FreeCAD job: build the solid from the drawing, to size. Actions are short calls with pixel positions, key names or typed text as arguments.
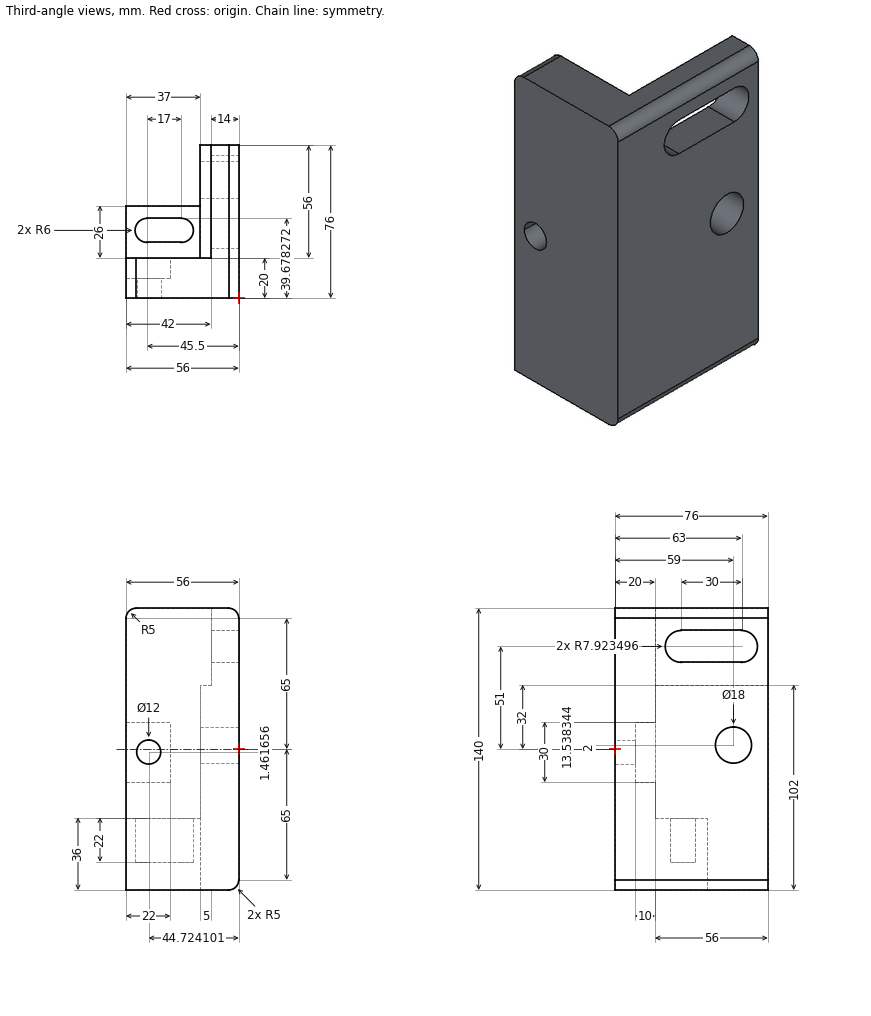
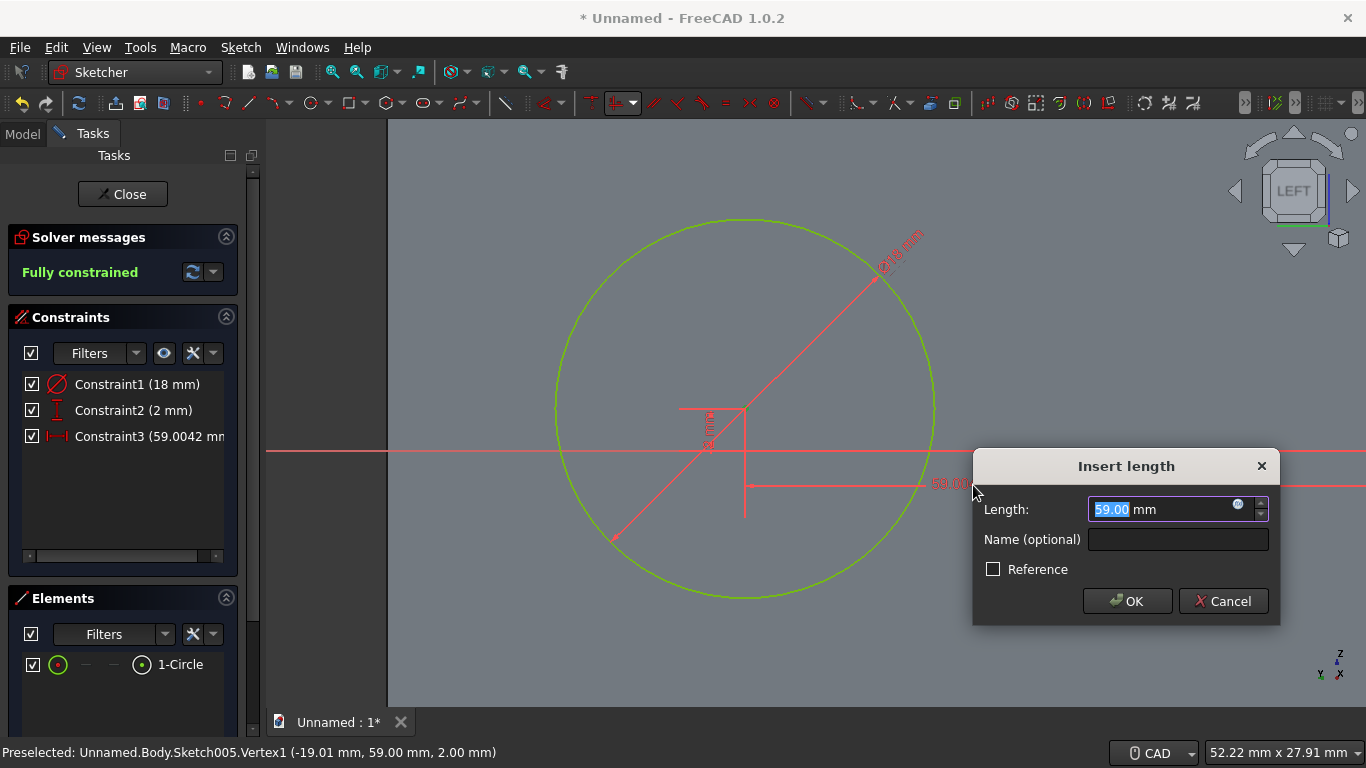
text(59)
key(Return)
key(Escape)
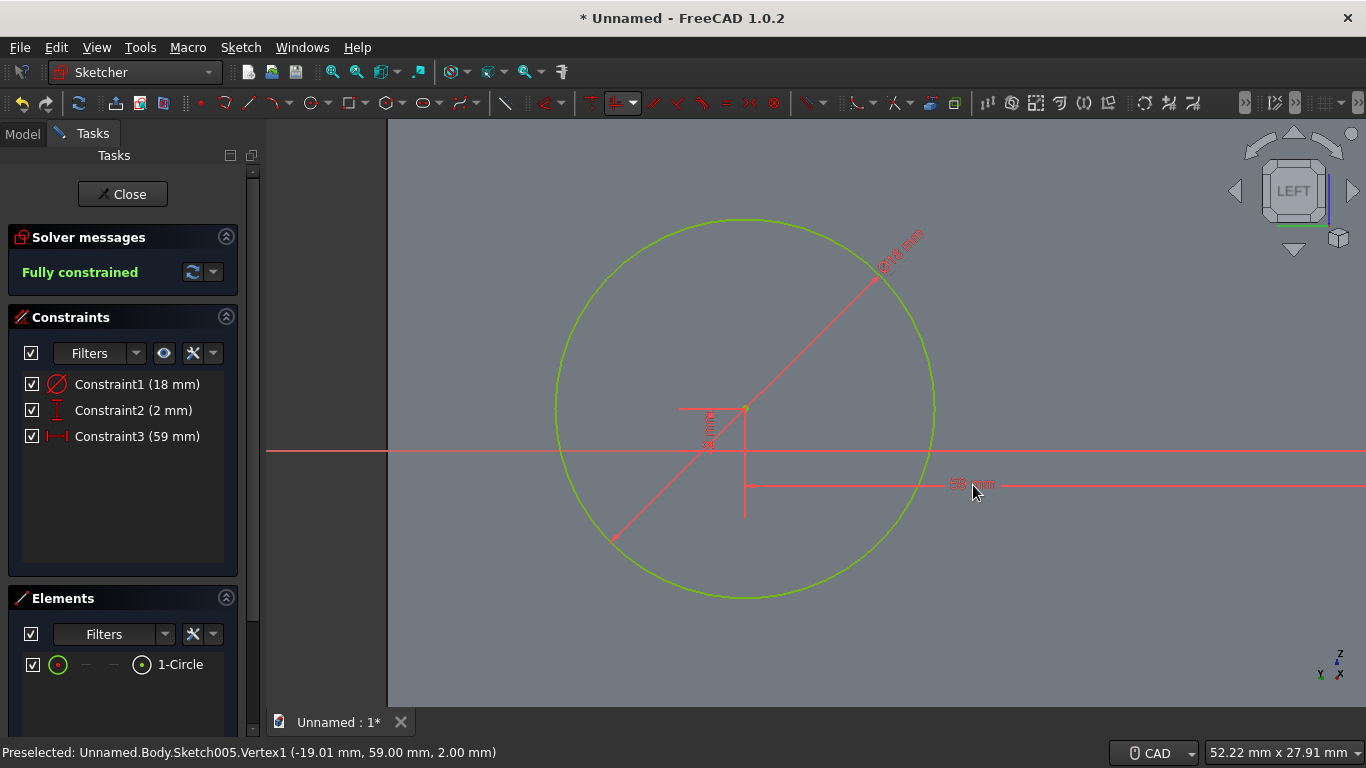
click(123, 194)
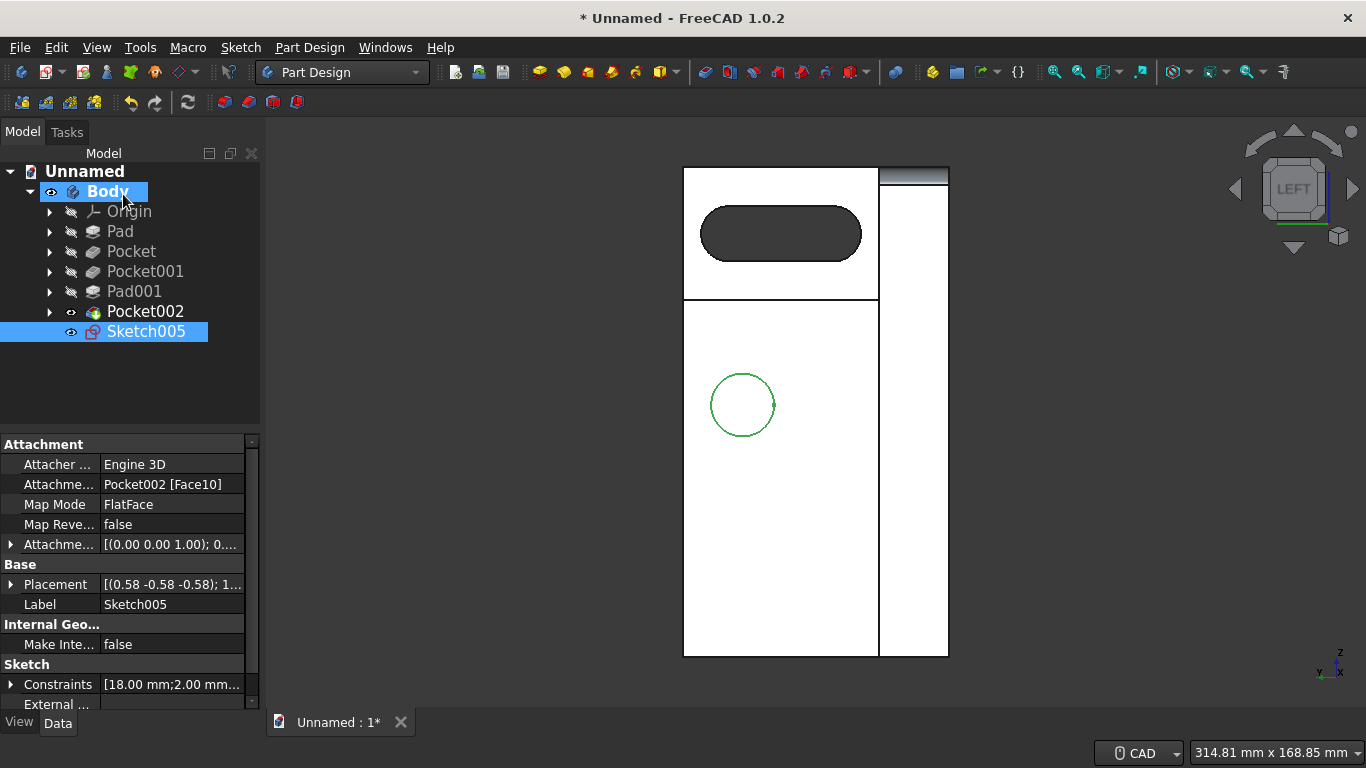
click(706, 72)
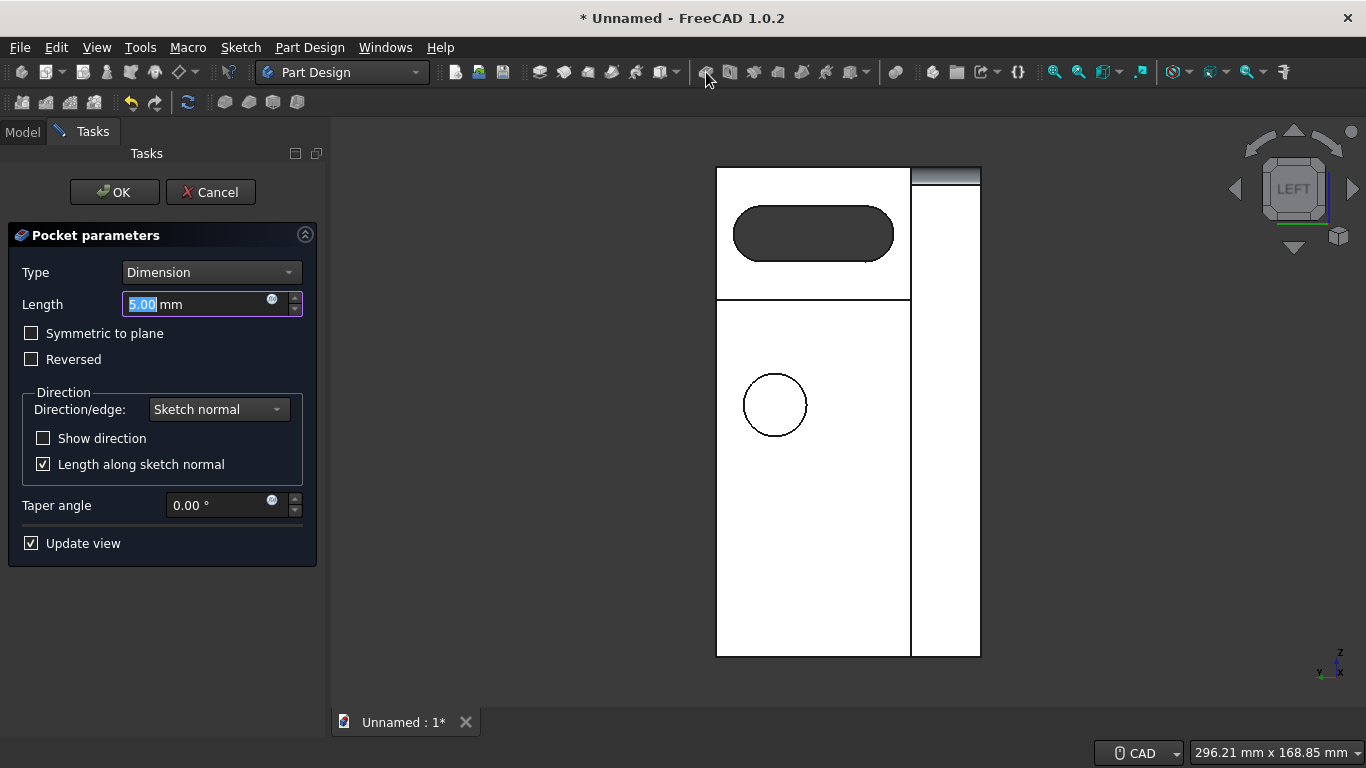
click(212, 272)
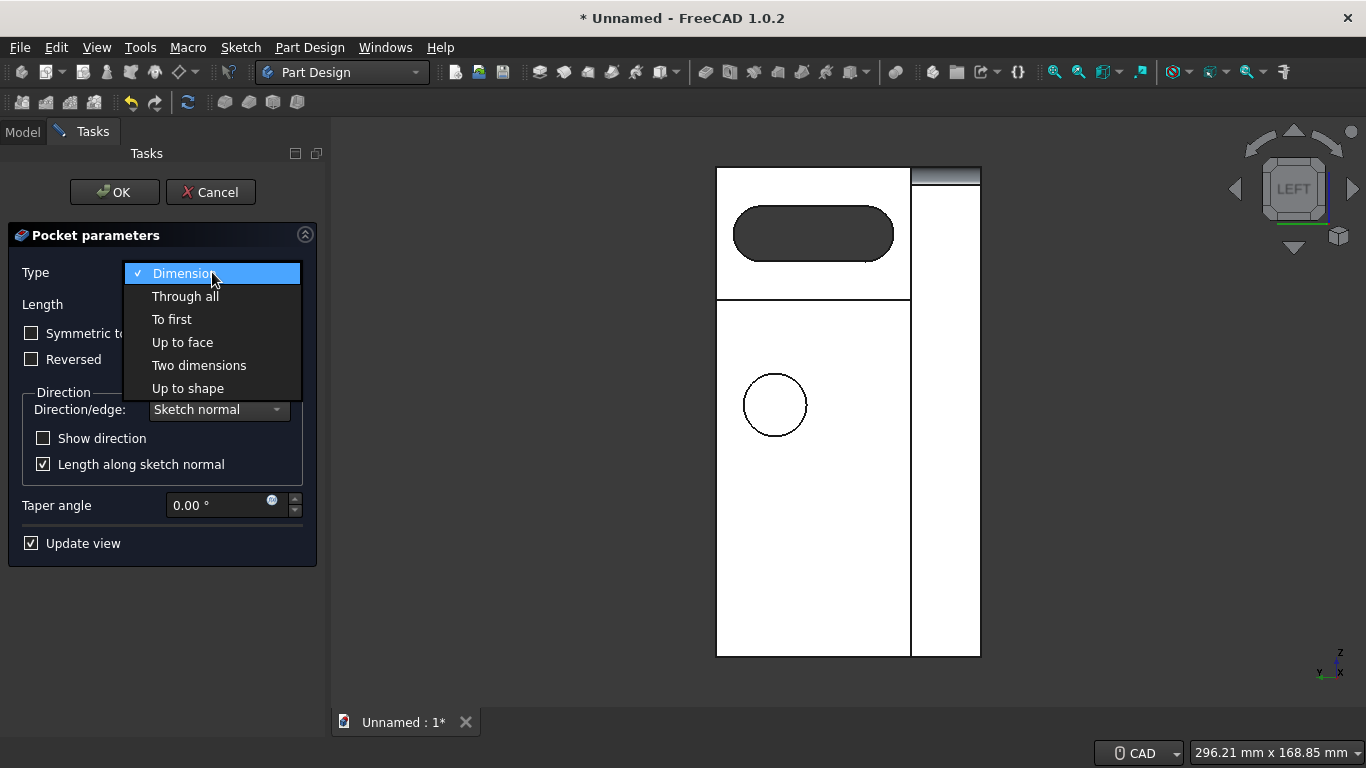
click(212, 296)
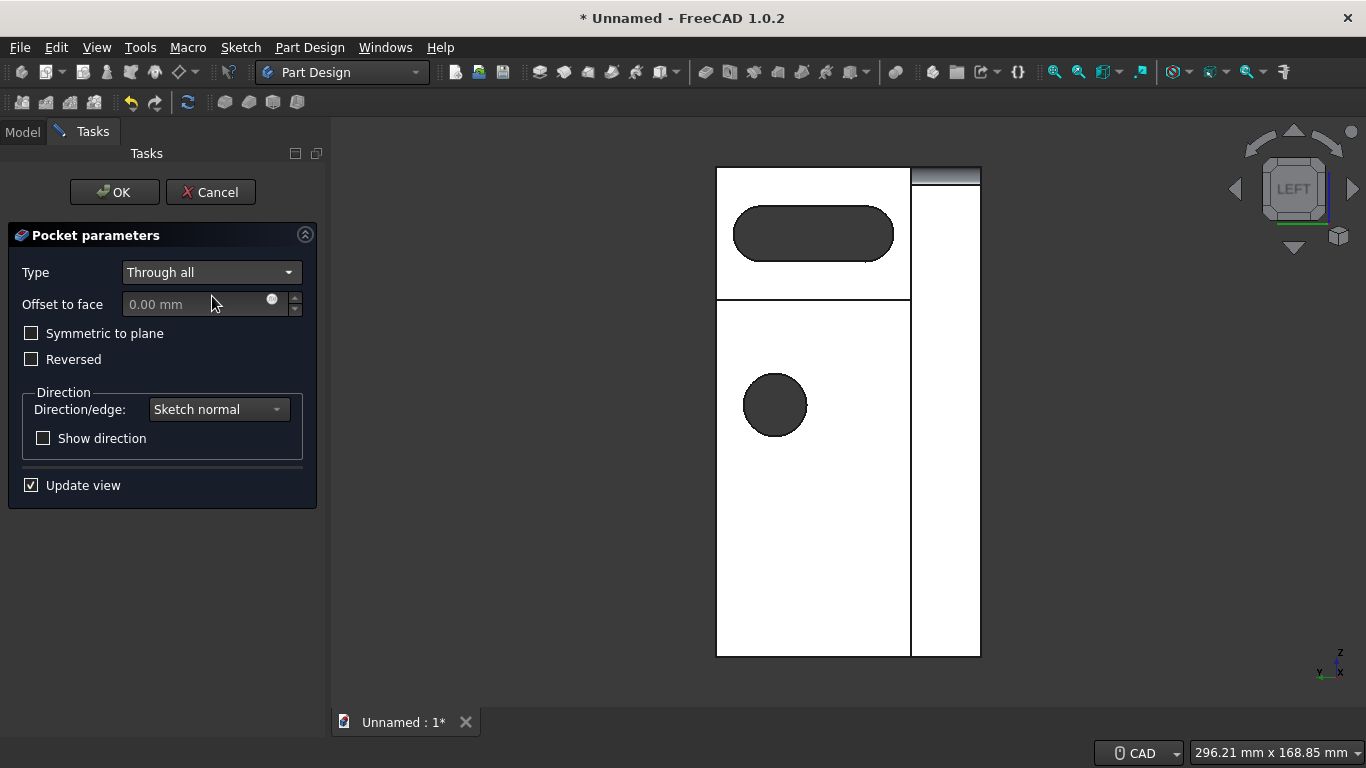
click(115, 192)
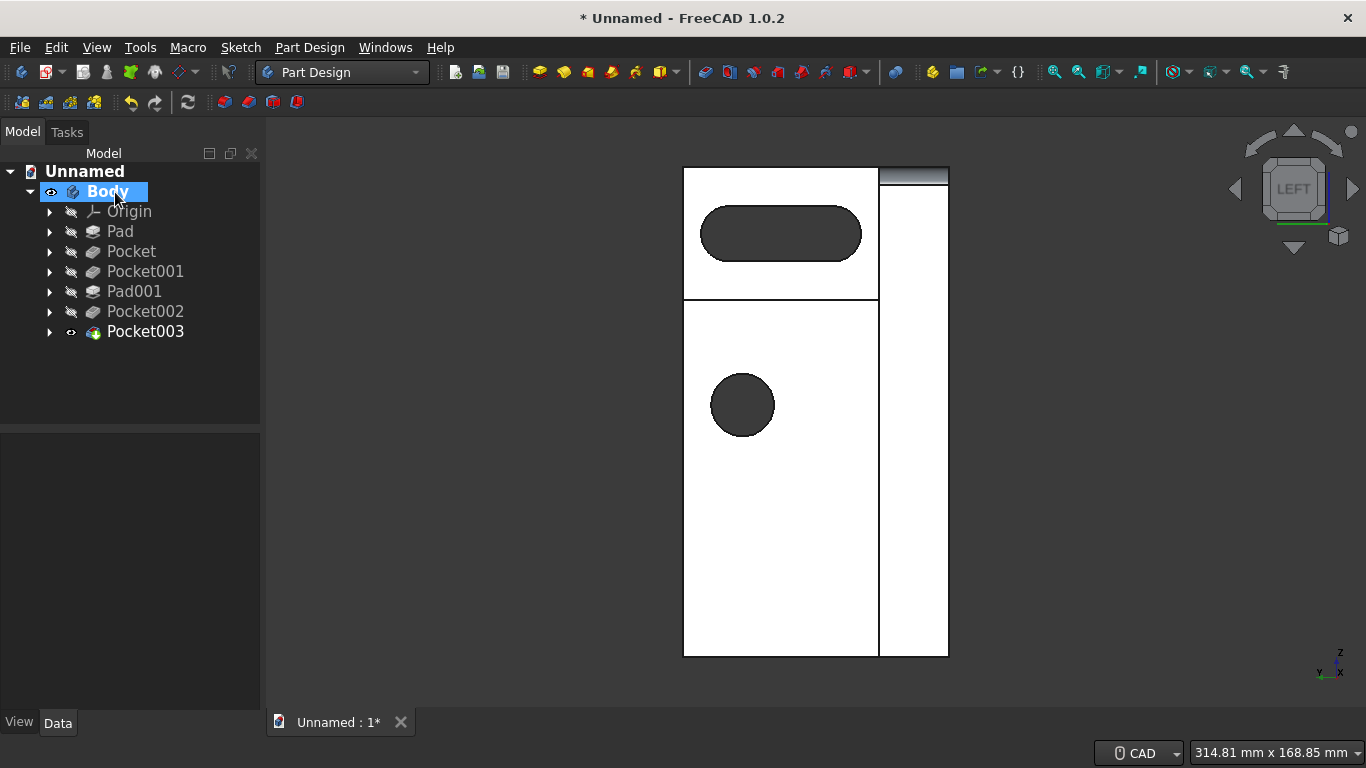
key(5)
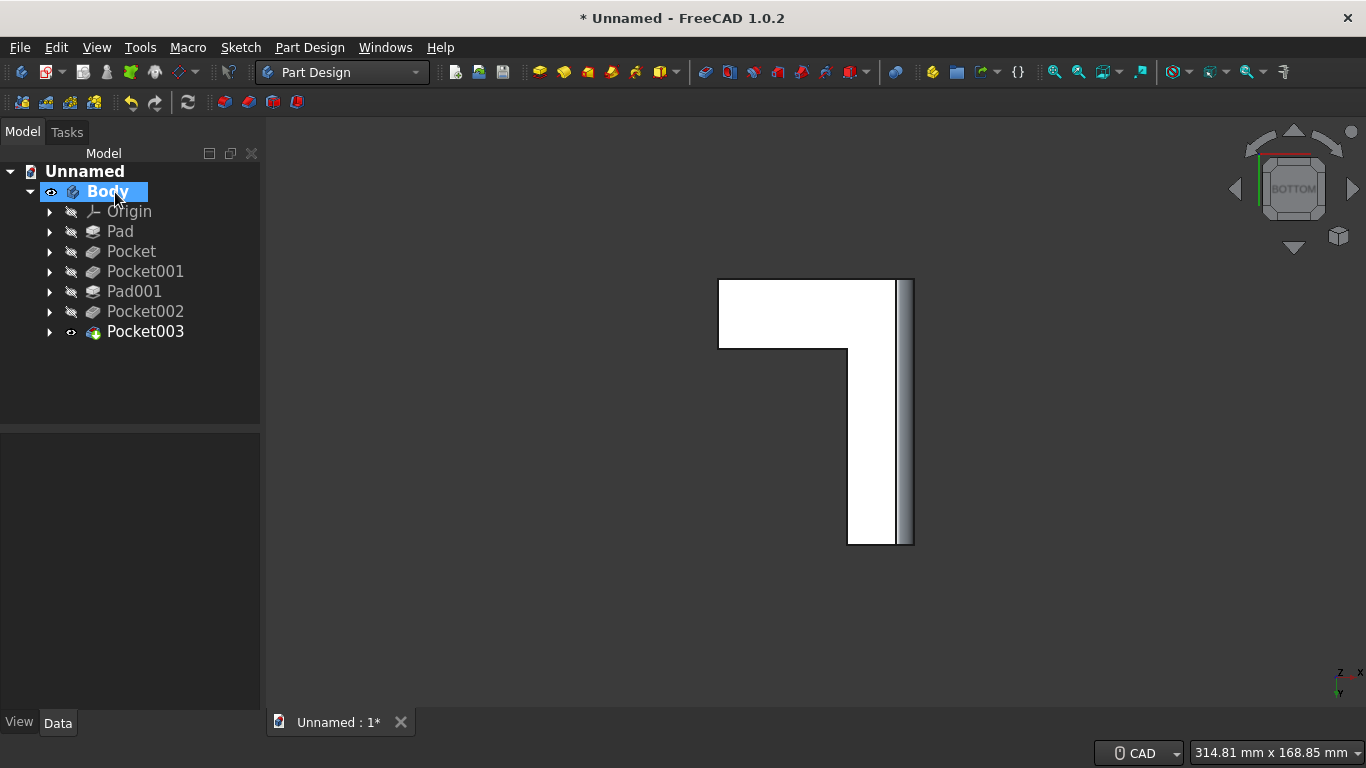
click(858, 297)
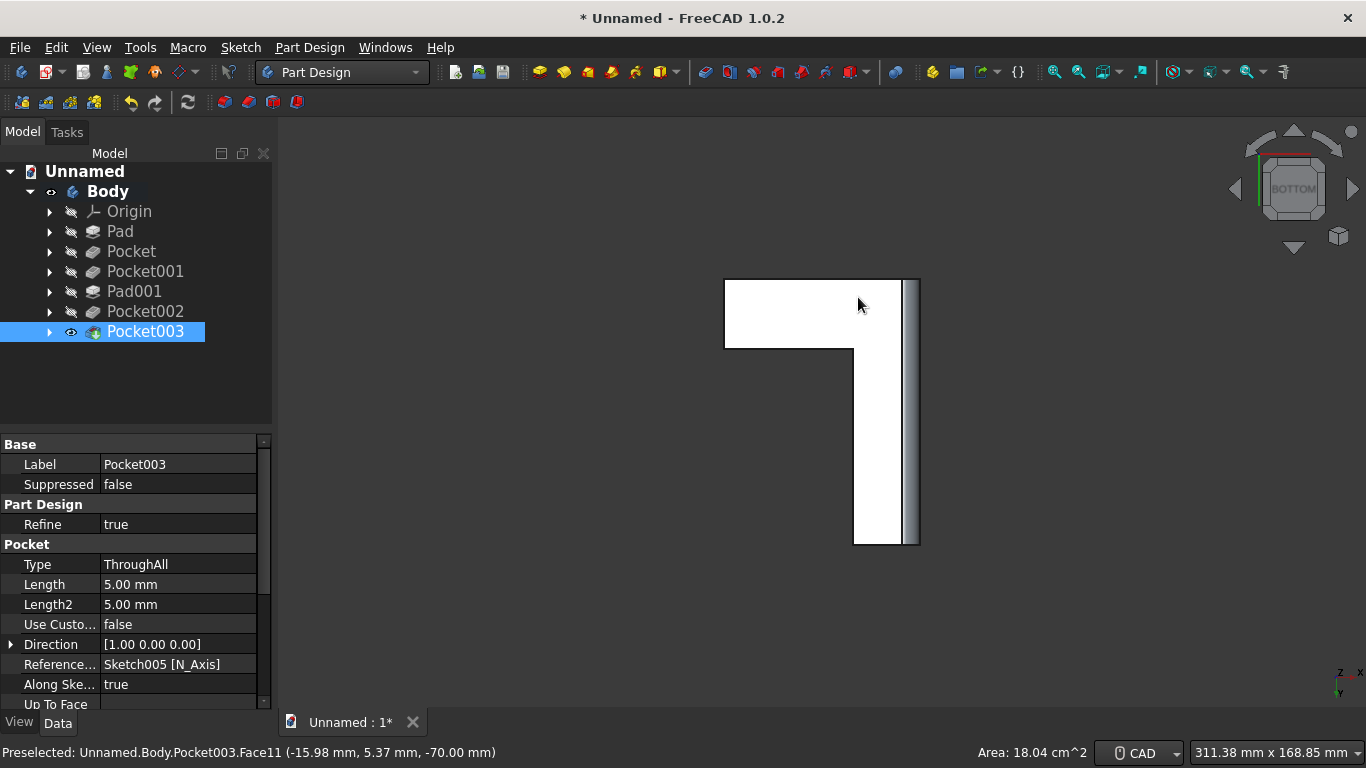
click(46, 72)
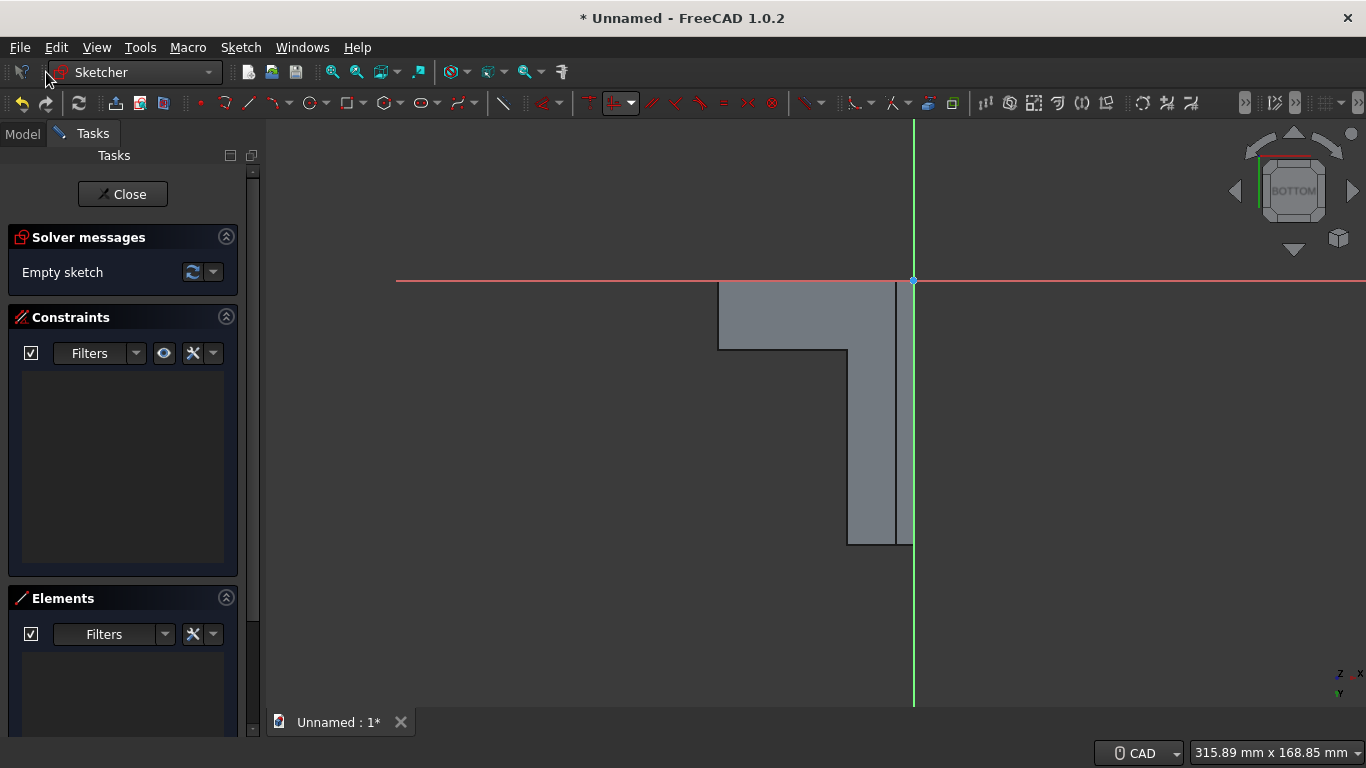
scroll(872, 318, up, 4)